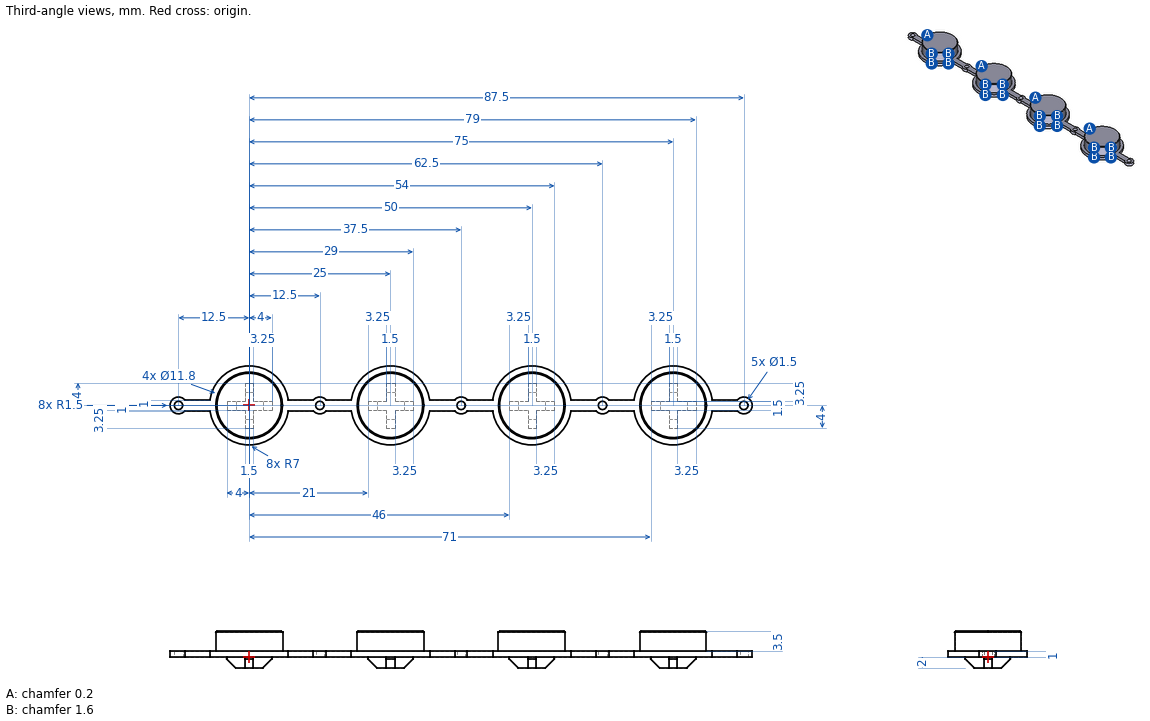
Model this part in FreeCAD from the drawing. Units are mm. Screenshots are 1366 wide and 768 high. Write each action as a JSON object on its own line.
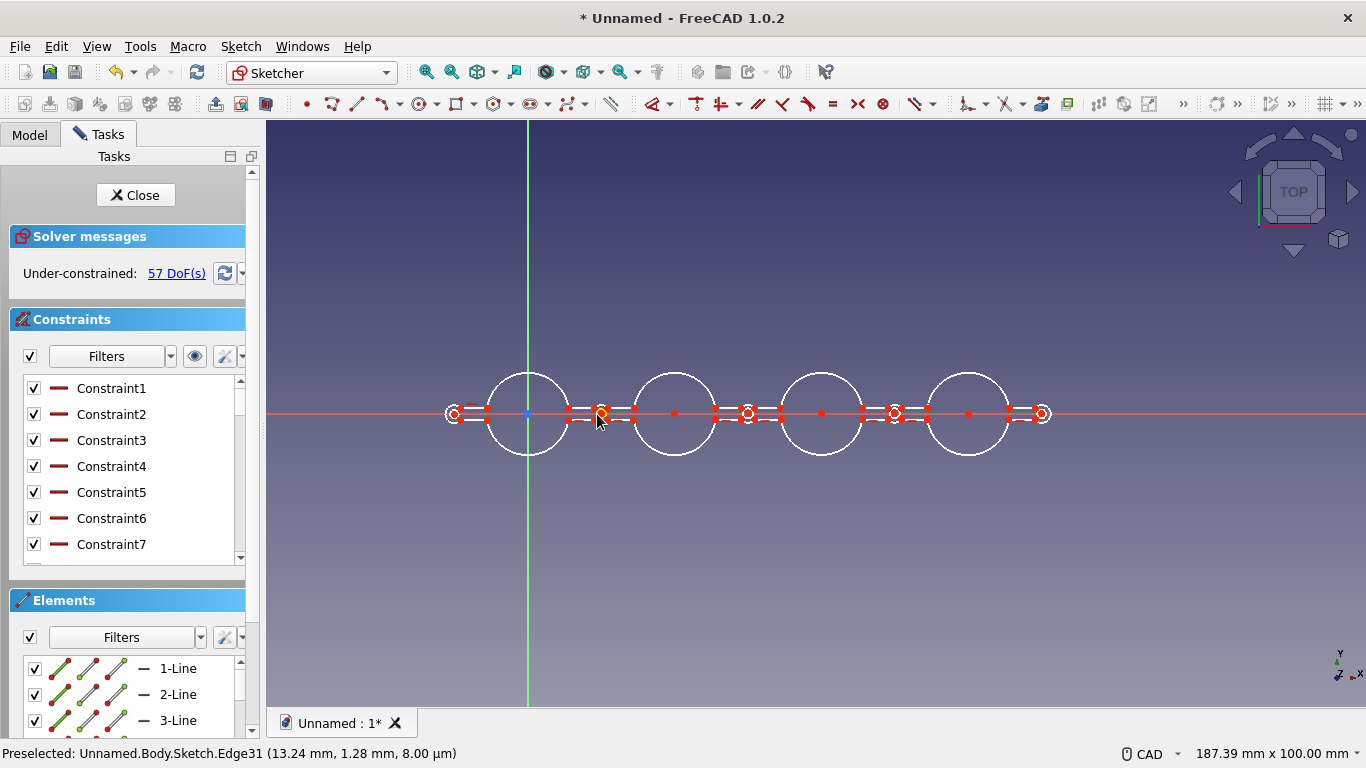
{"action": "left_click", "coordinate": [550, 449]}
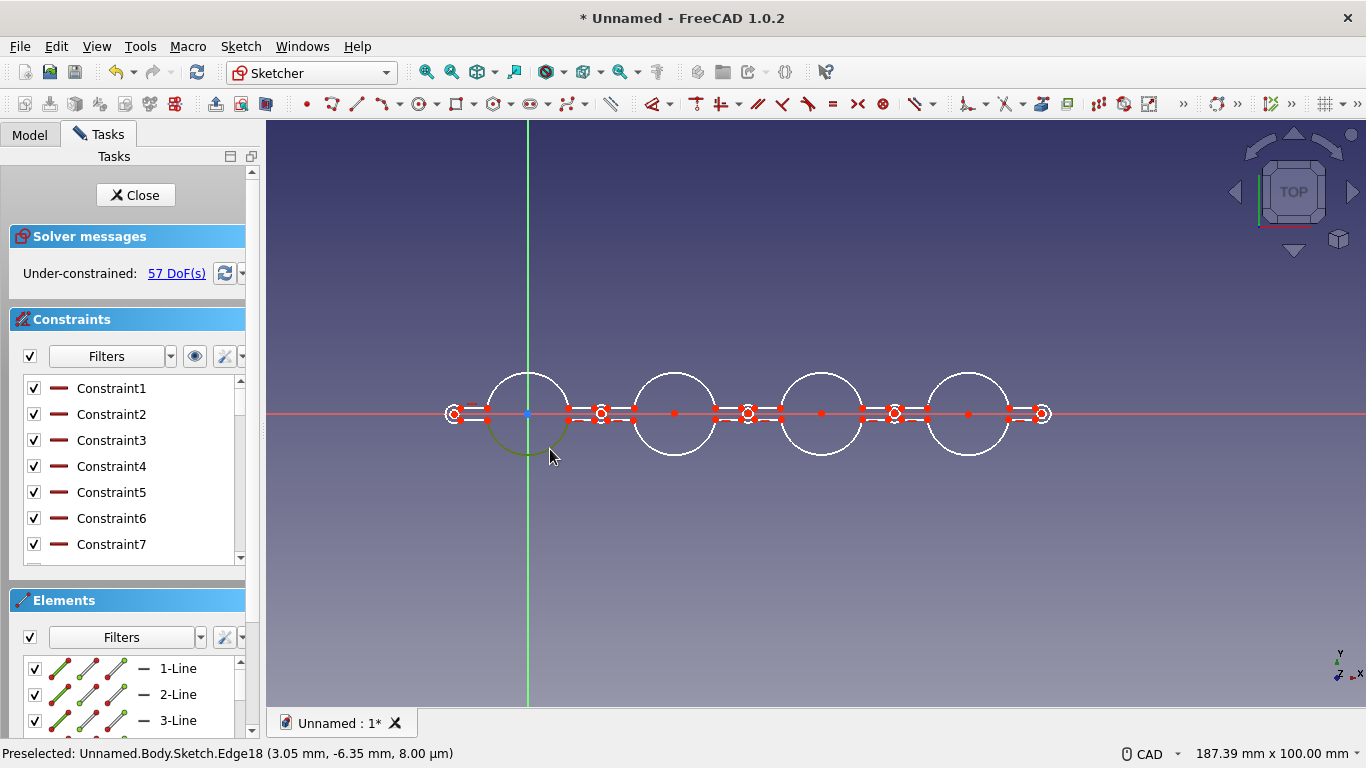
{"action": "left_click", "coordinate": [550, 379]}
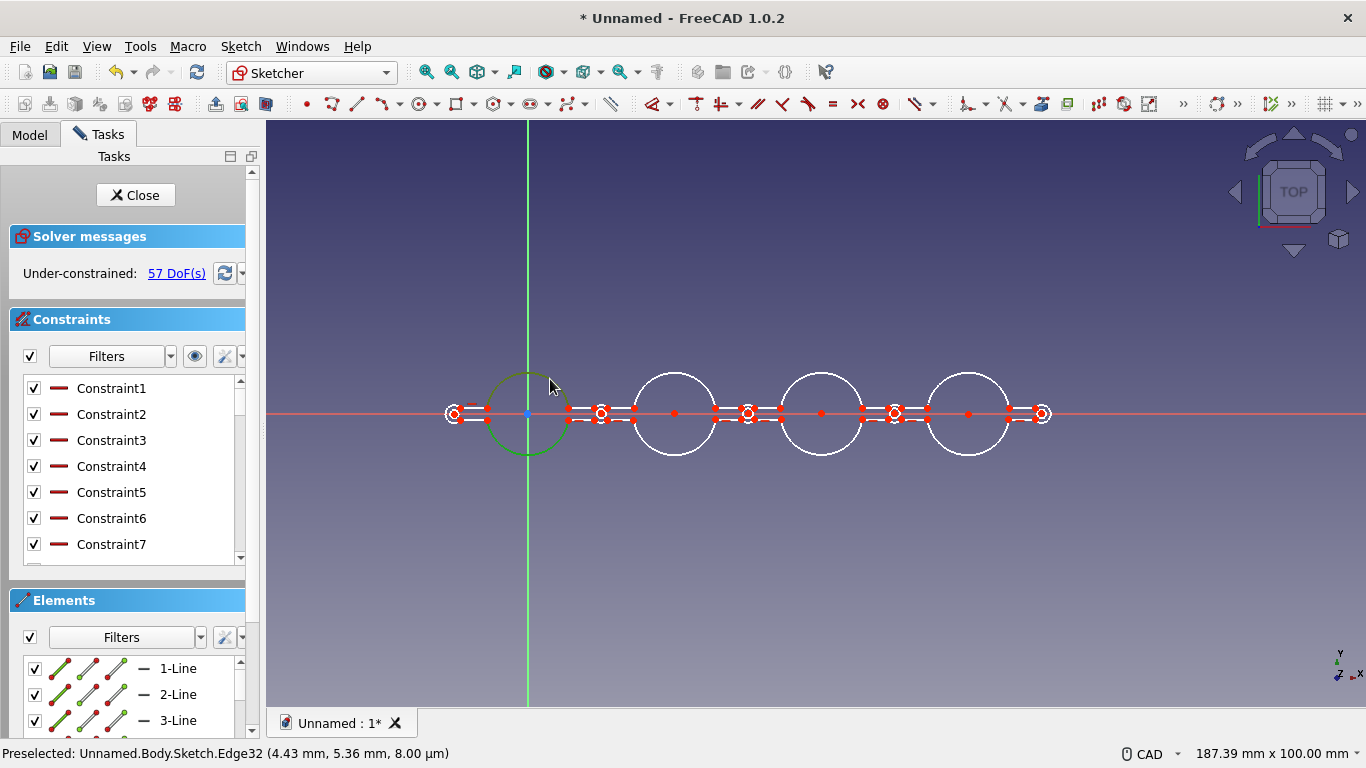
{"action": "key", "text": "c"}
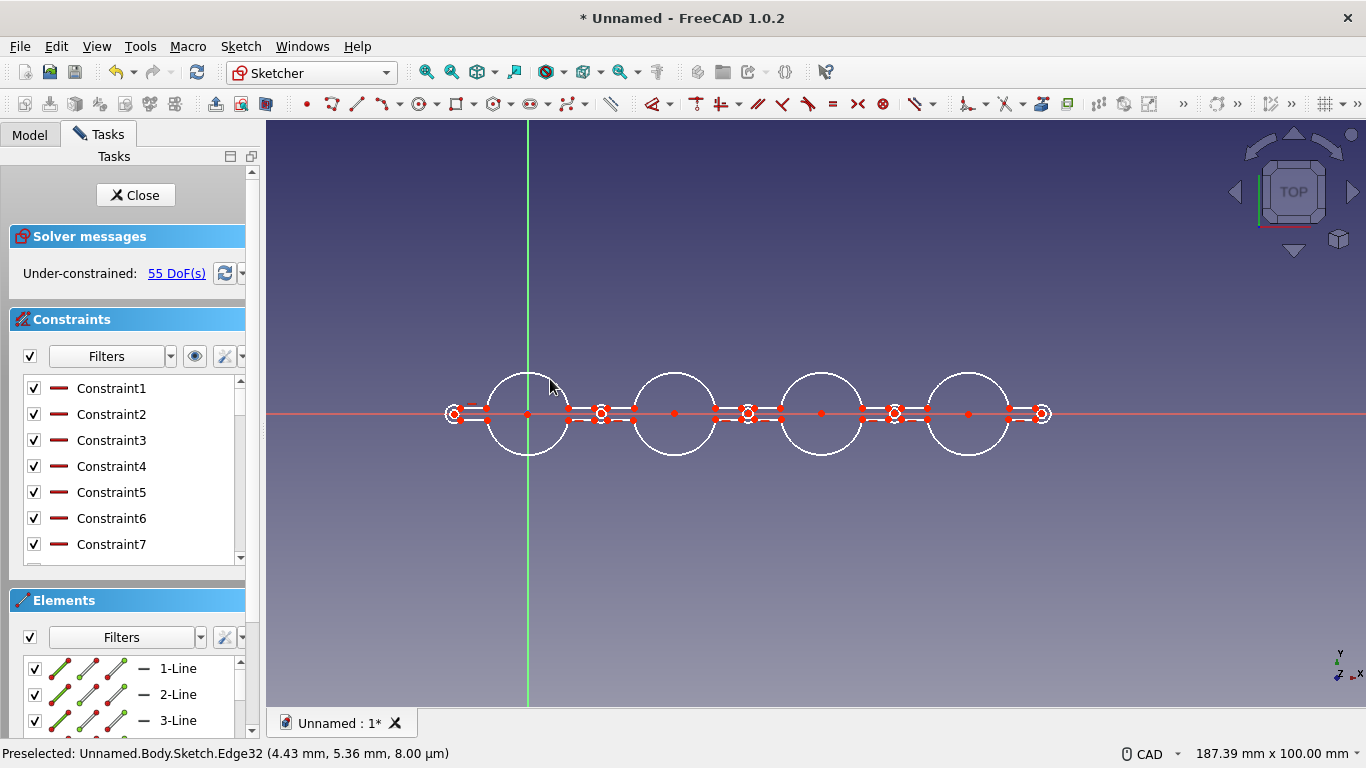
{"action": "scroll", "coordinate": [528, 414], "scroll_direction": "up", "scroll_amount": 12}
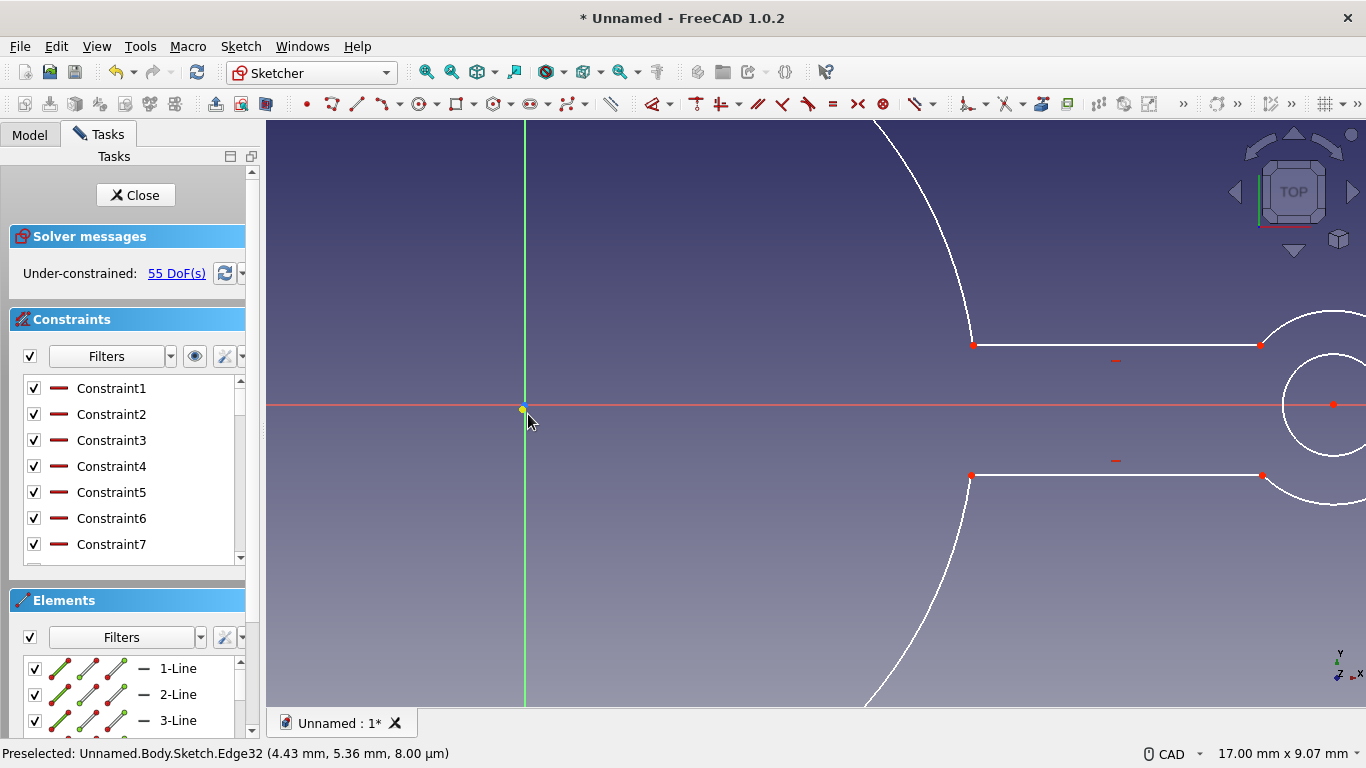
{"action": "left_click_drag", "start_coordinate": [513, 395], "coordinate": [535, 419]}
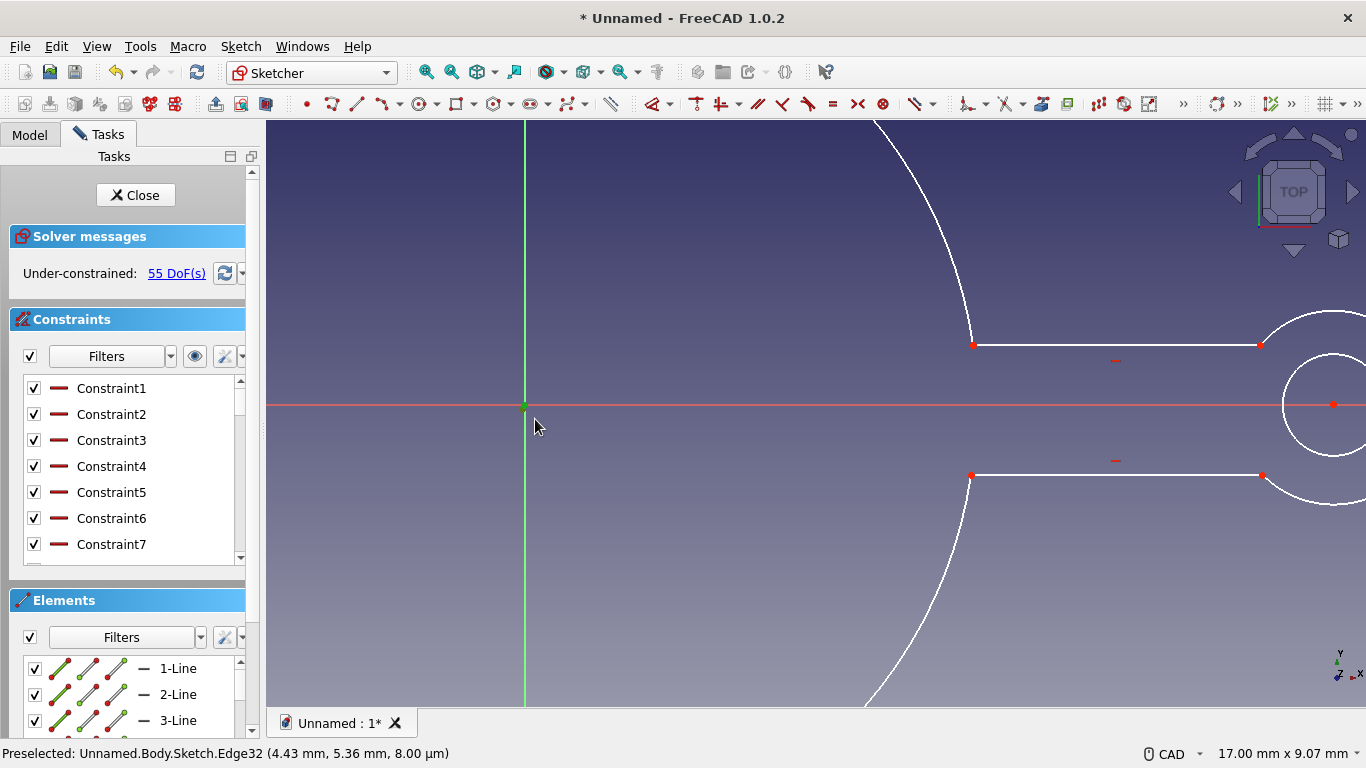
{"action": "key", "text": "c"}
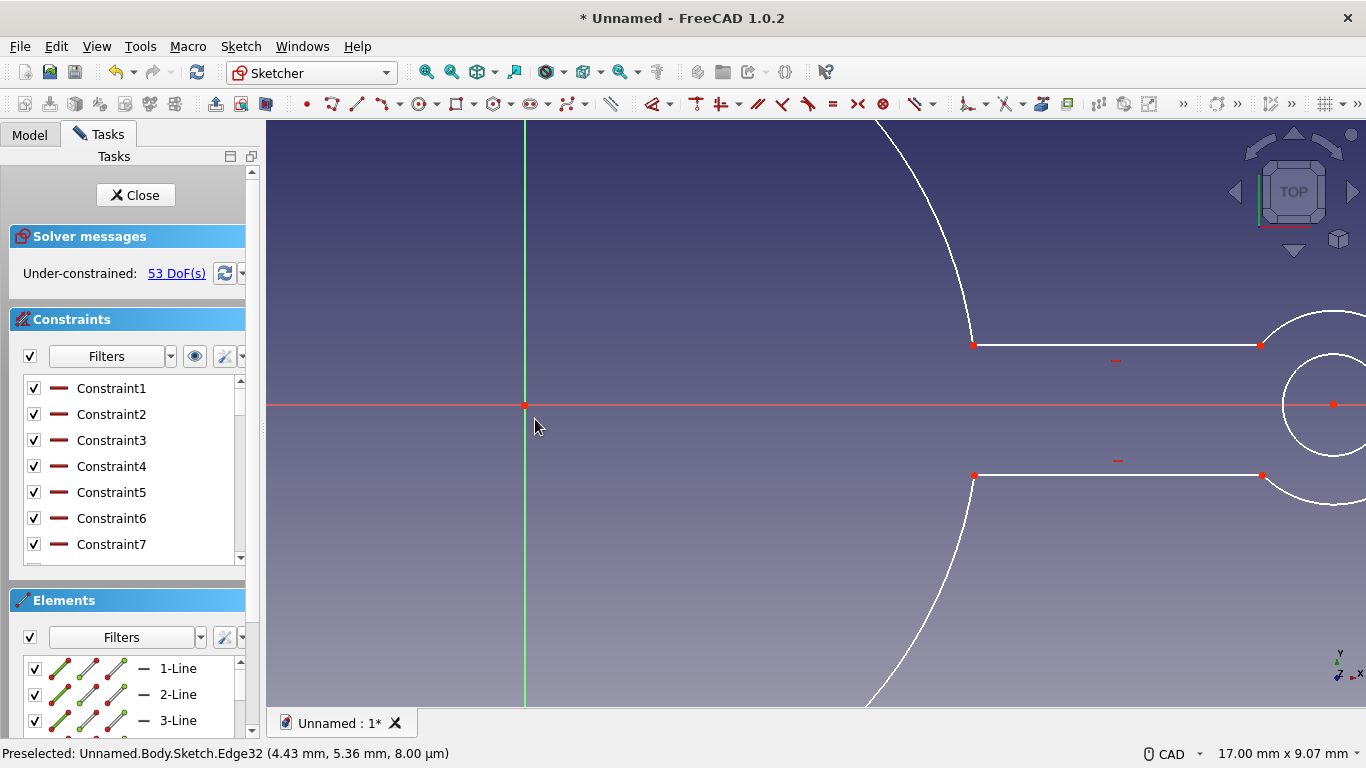
{"action": "scroll", "coordinate": [528, 414], "scroll_direction": "down", "scroll_amount": 12}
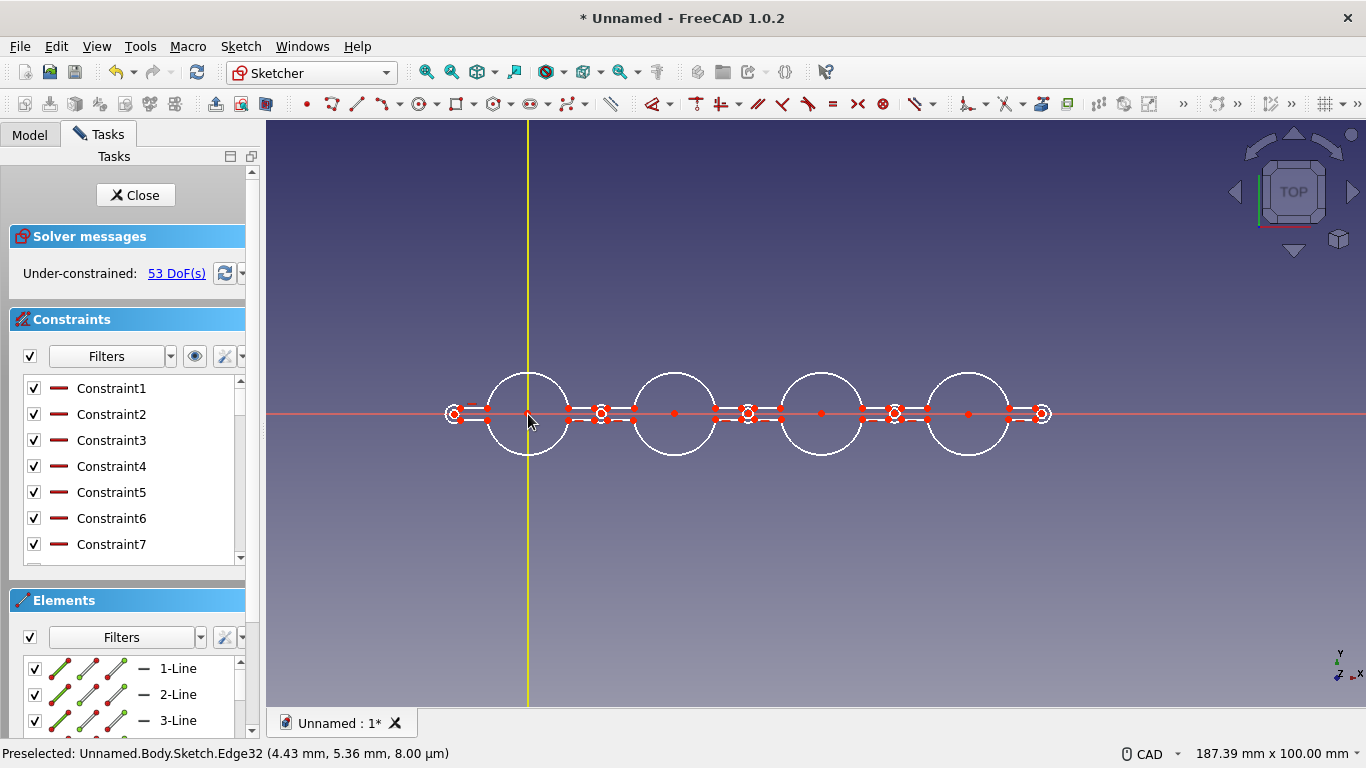
{"action": "scroll", "coordinate": [449, 407], "scroll_direction": "up", "scroll_amount": 6}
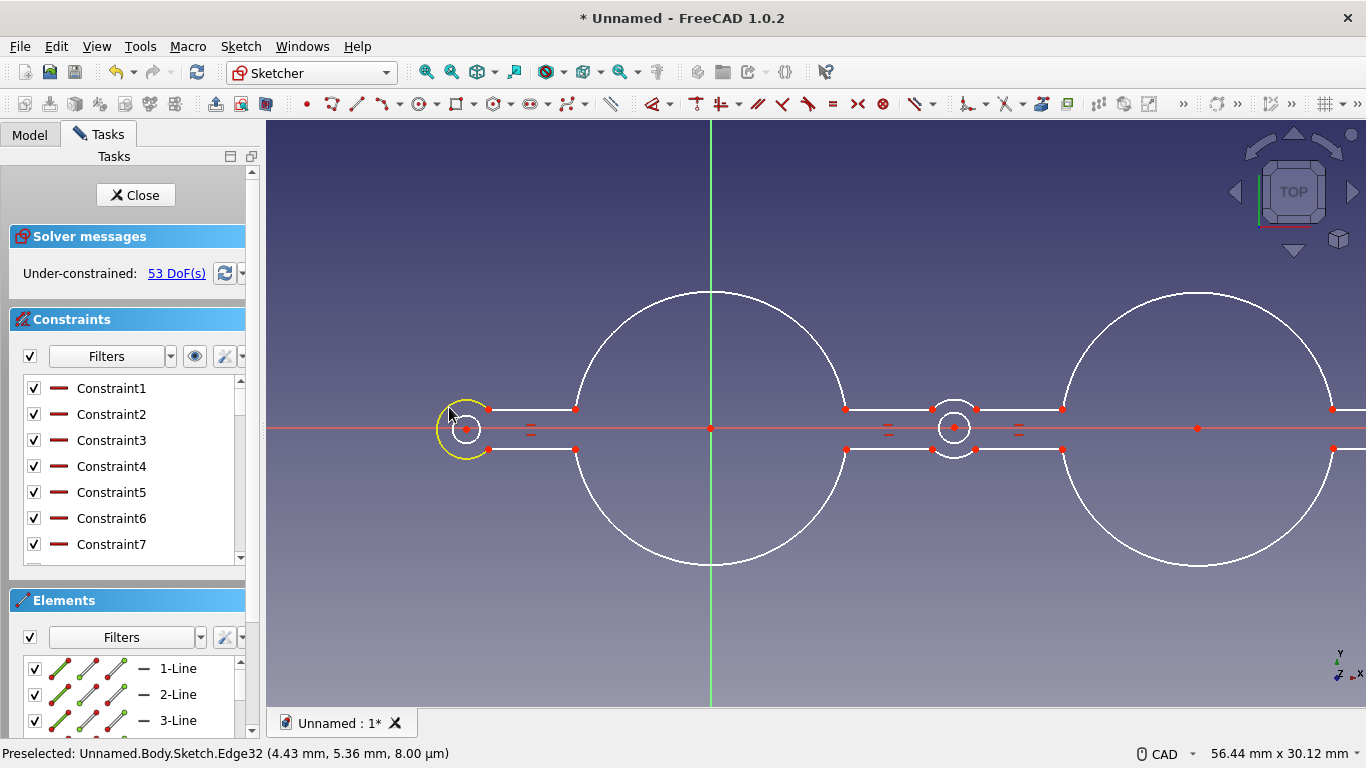
{"action": "left_click", "coordinate": [450, 405]}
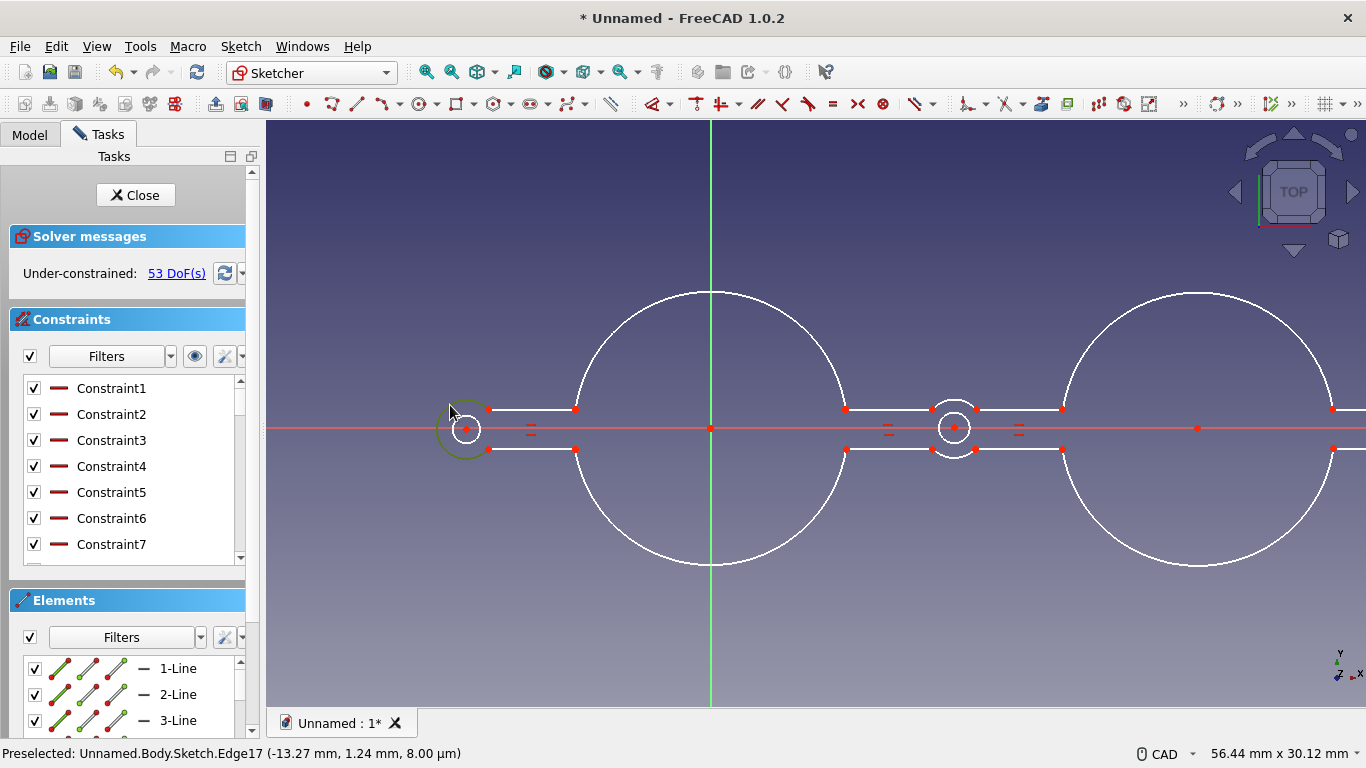
{"action": "left_click", "coordinate": [945, 456]}